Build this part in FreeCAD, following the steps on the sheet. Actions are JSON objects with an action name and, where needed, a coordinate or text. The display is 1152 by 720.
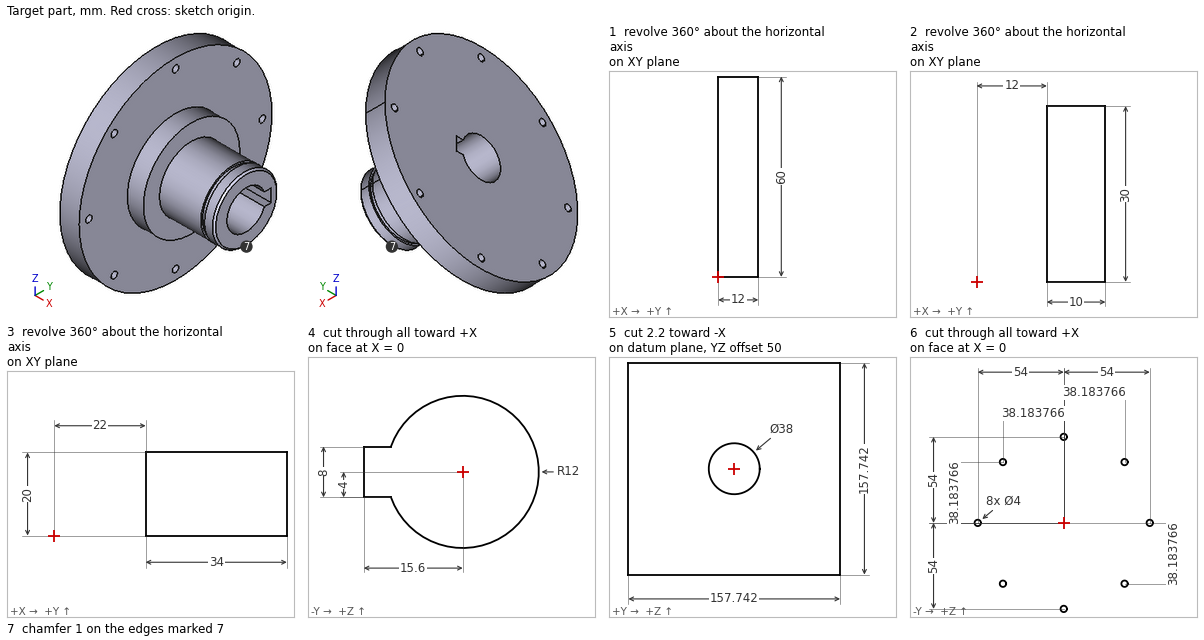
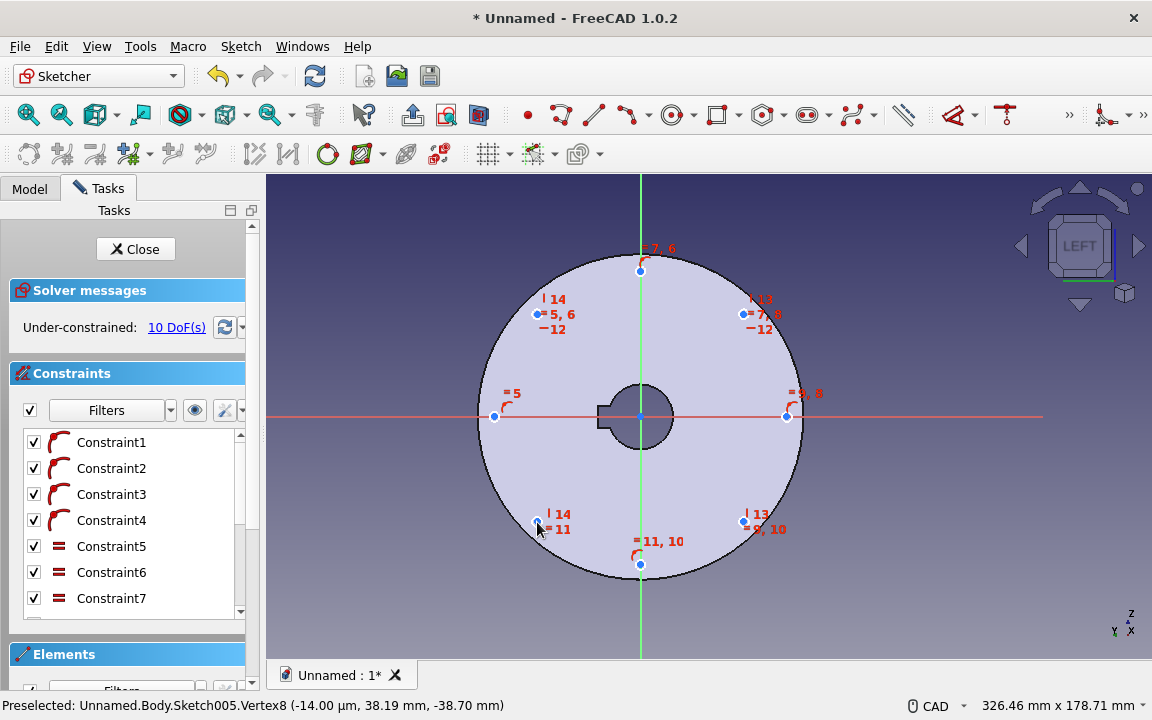
{"action": "scroll", "coordinate": [744, 522], "scroll_direction": "up", "scroll_amount": 4}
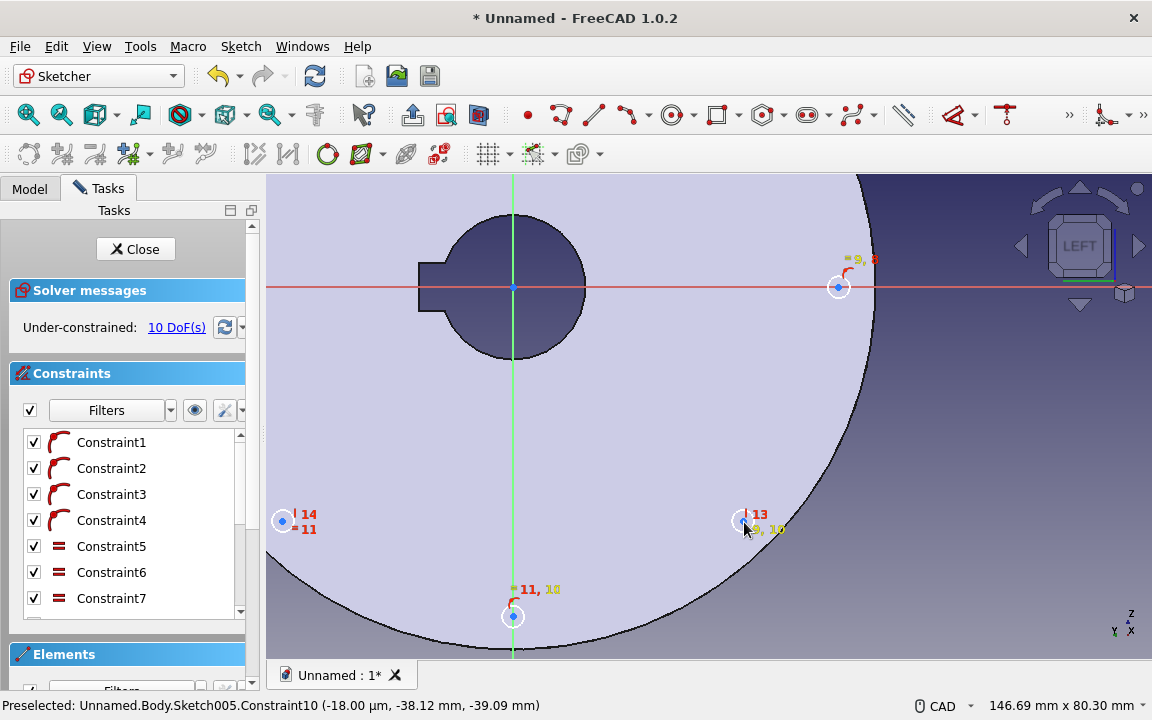
{"action": "scroll", "coordinate": [743, 521], "scroll_direction": "up", "scroll_amount": 4}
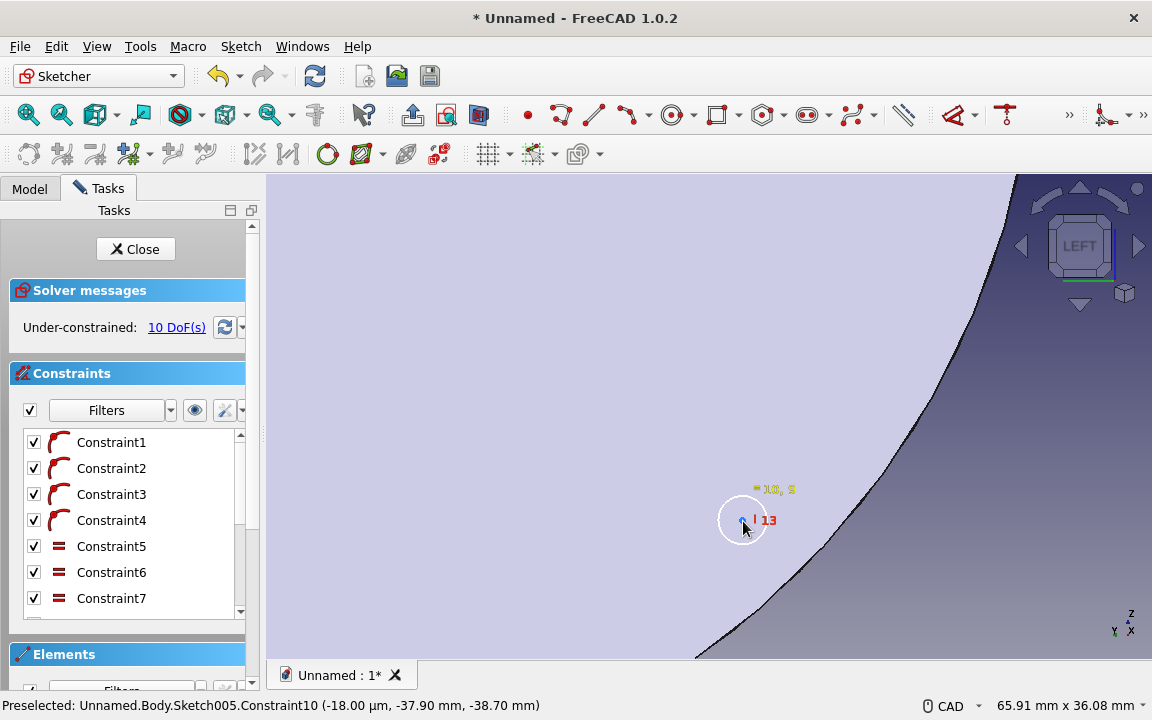
{"action": "left_click", "coordinate": [743, 520]}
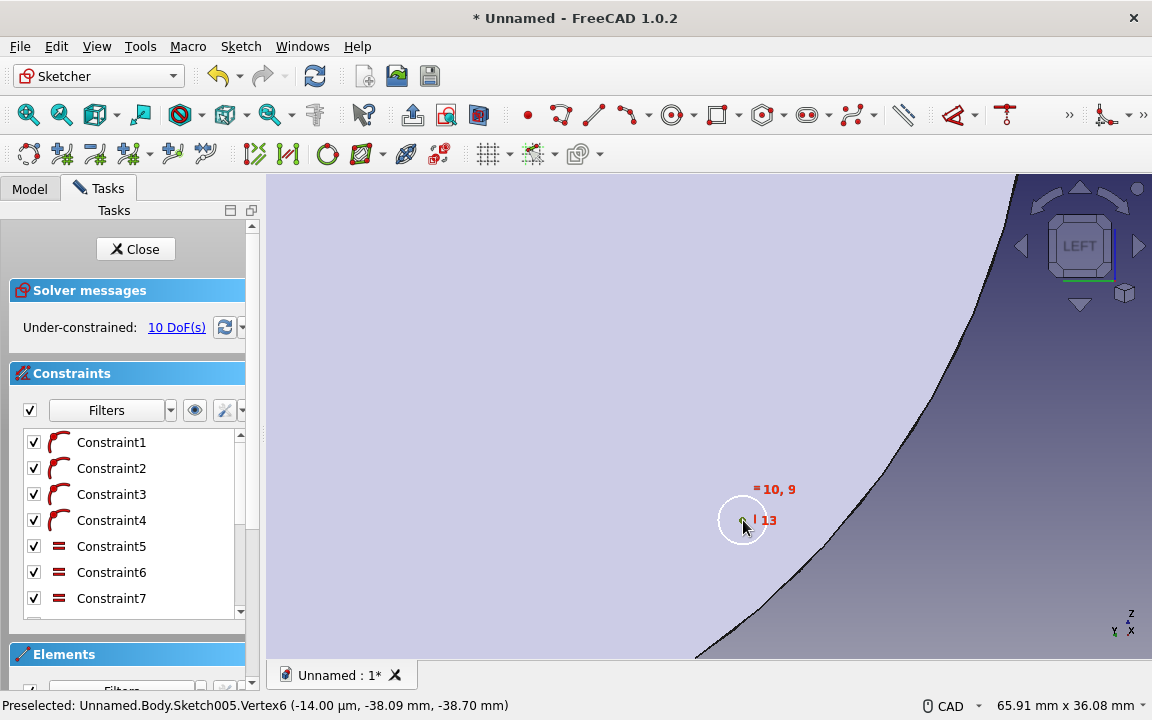
{"action": "scroll", "coordinate": [744, 522], "scroll_direction": "down", "scroll_amount": 8}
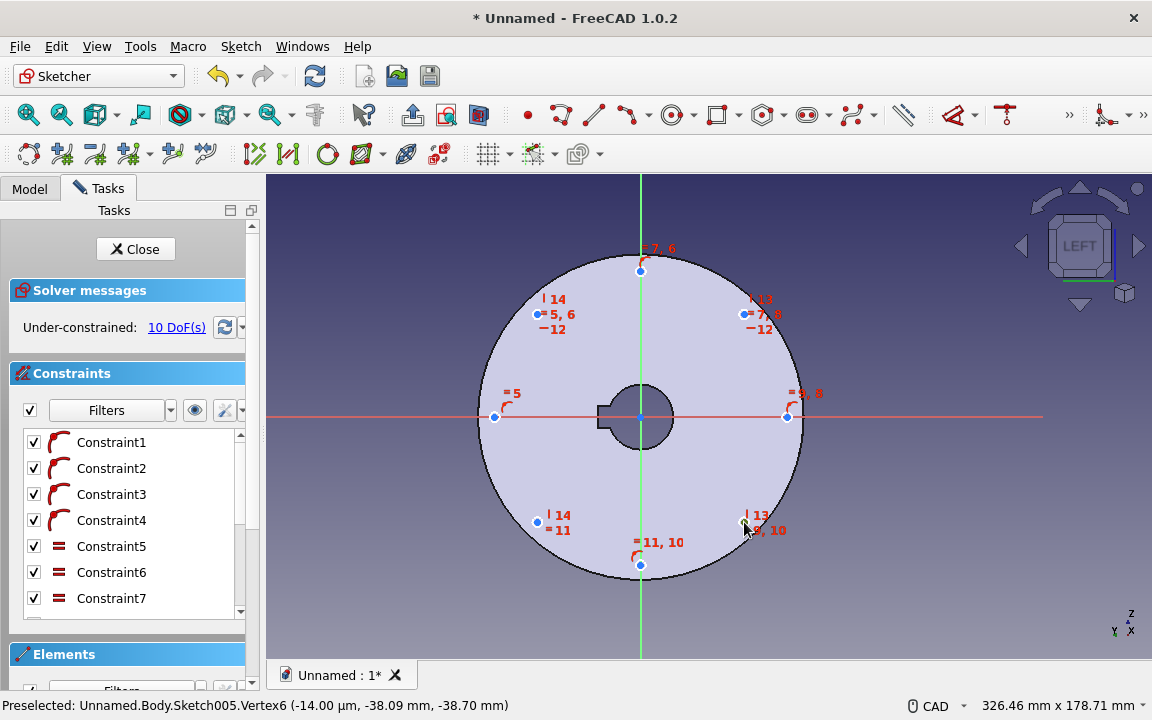
{"action": "left_click", "coordinate": [537, 522]}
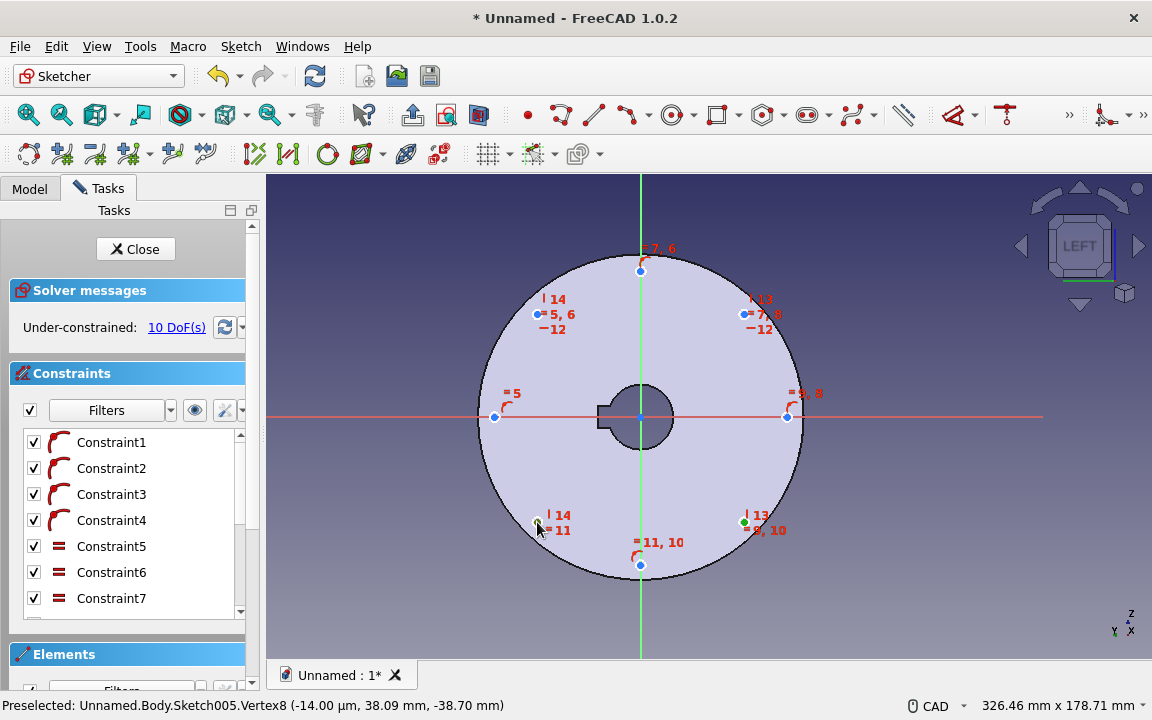
{"action": "key", "text": "h"}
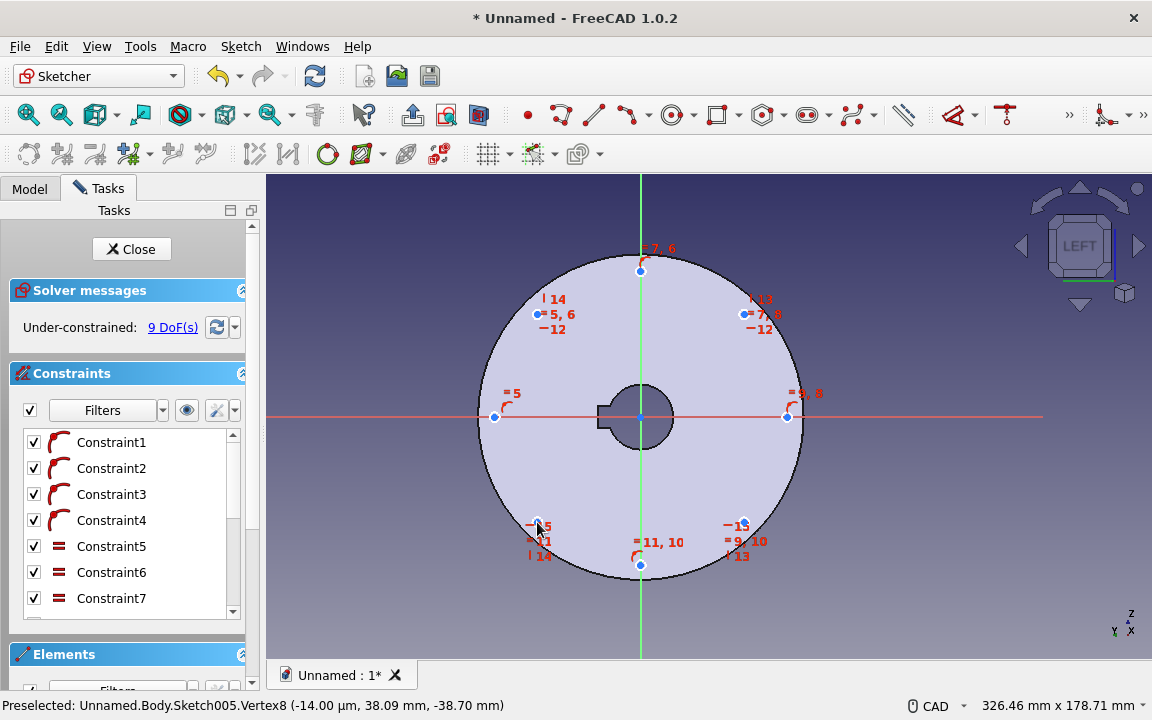
{"action": "left_click", "coordinate": [952, 116]}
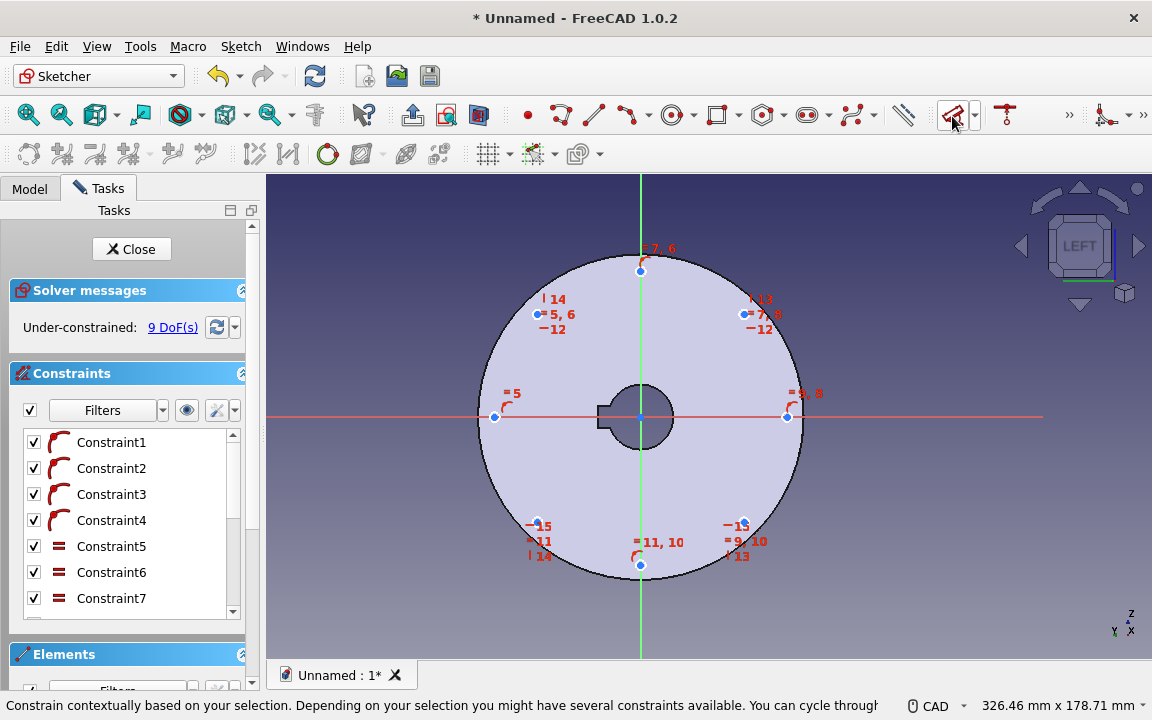
{"action": "scroll", "coordinate": [490, 417], "scroll_direction": "up", "scroll_amount": 7}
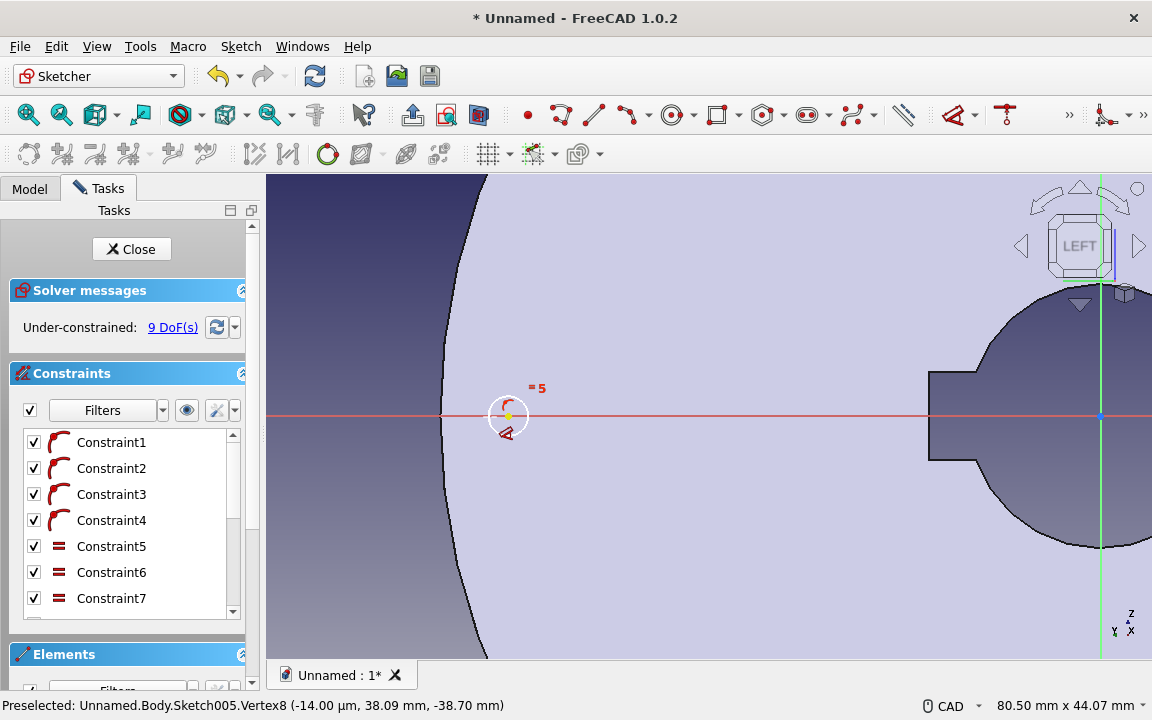
{"action": "left_click", "coordinate": [488, 416]}
{"action": "left_click", "coordinate": [463, 391]}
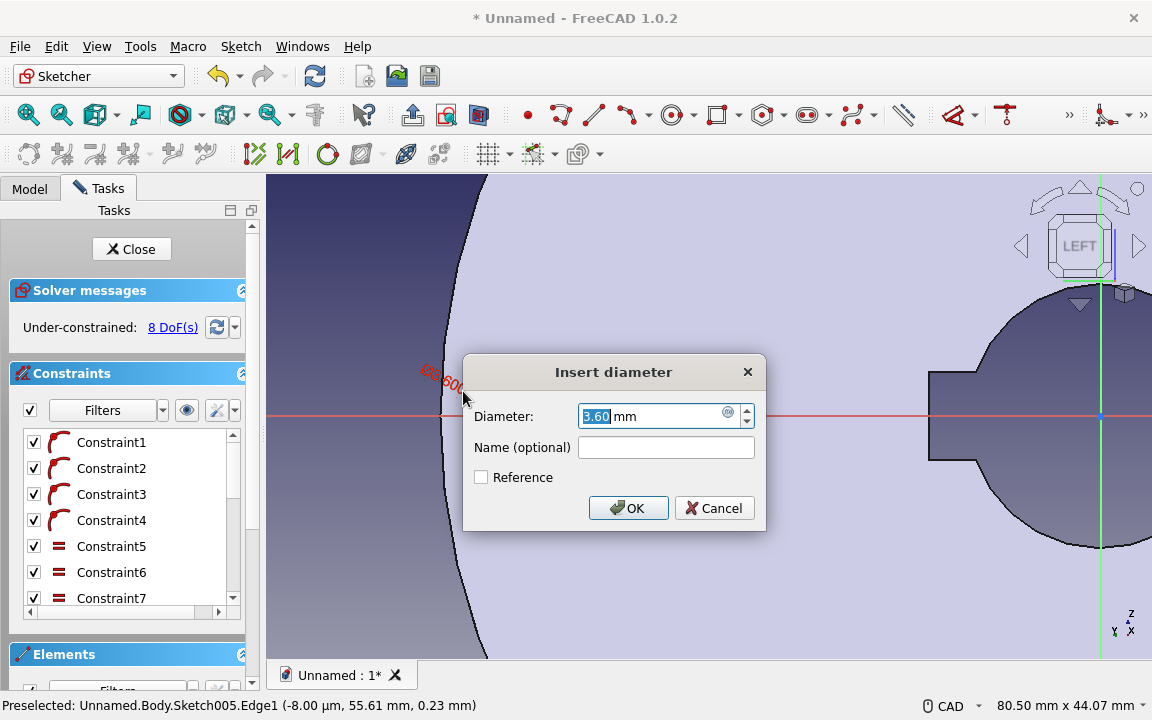
{"action": "type", "text": "4"}
{"action": "key", "text": "Return"}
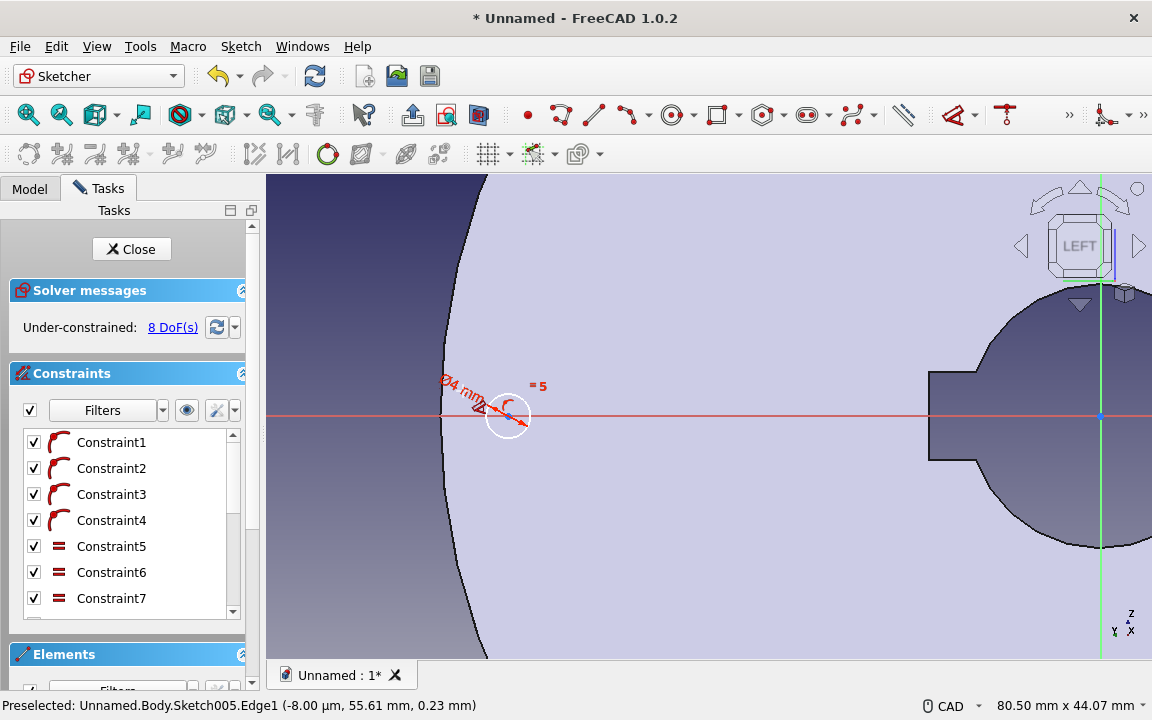
{"action": "scroll", "coordinate": [490, 417], "scroll_direction": "down", "scroll_amount": 7}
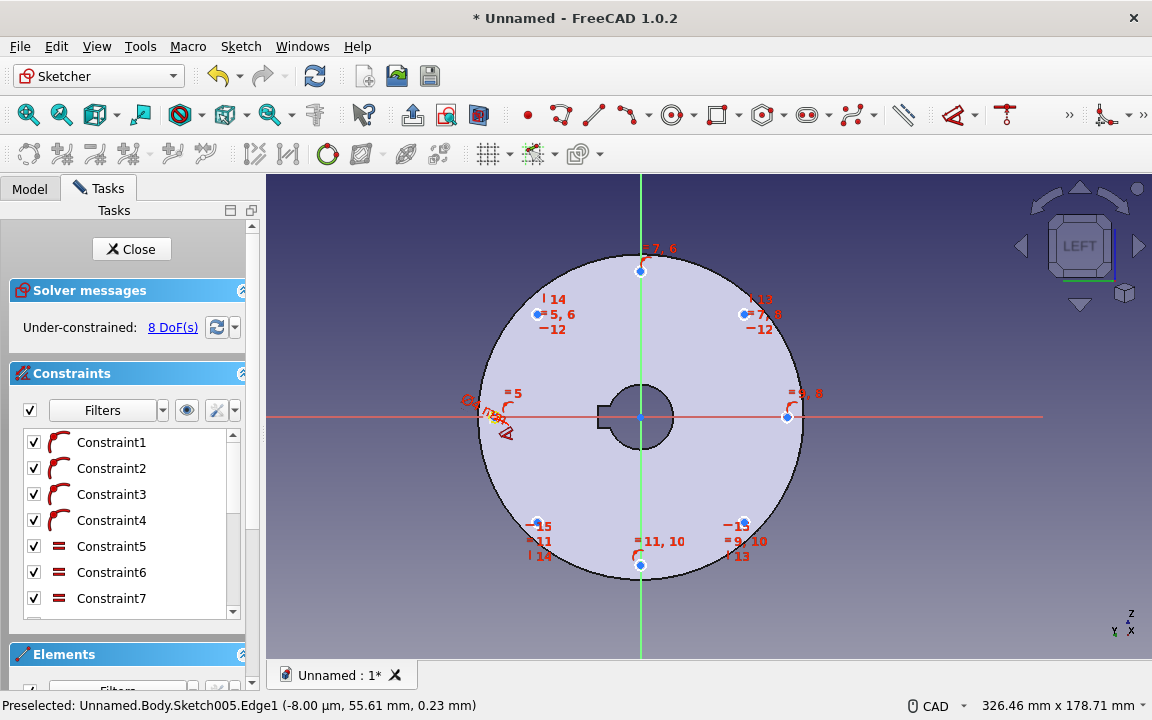
{"action": "left_click", "coordinate": [495, 417]}
{"action": "left_click", "coordinate": [568, 451]}